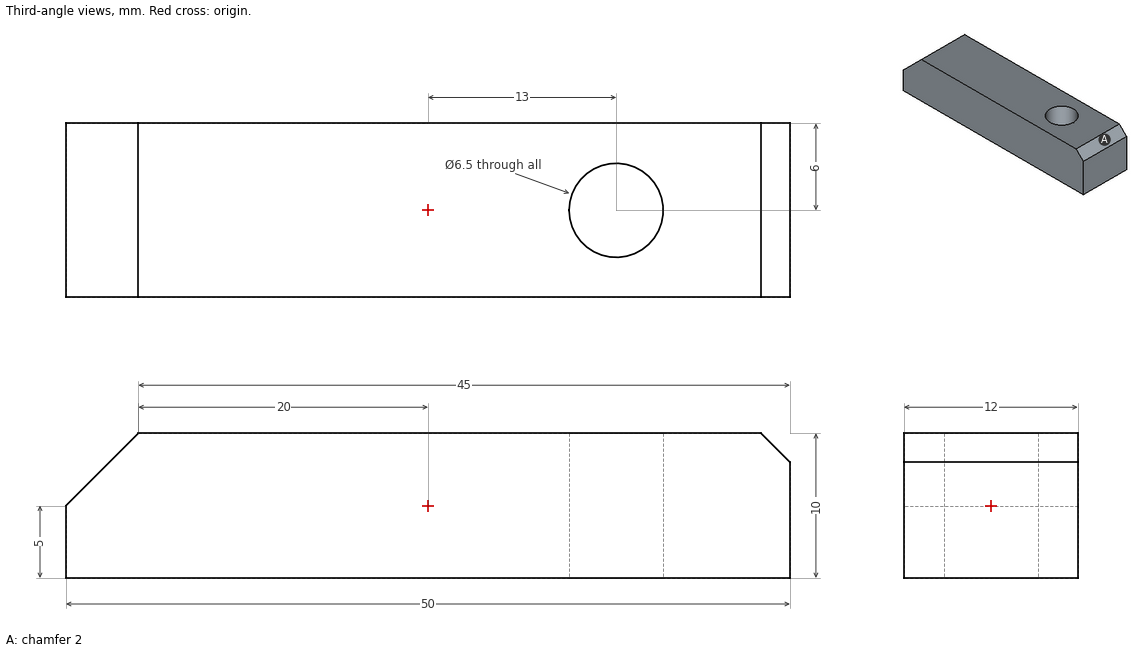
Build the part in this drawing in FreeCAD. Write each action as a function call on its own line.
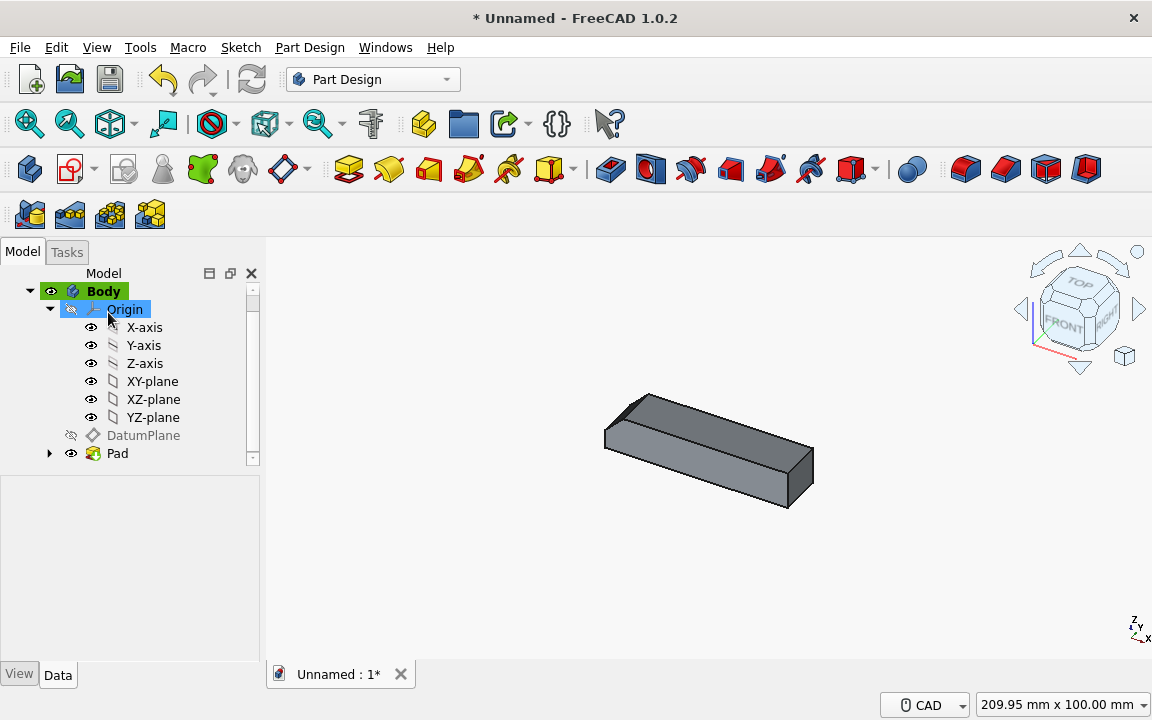
click(30, 124)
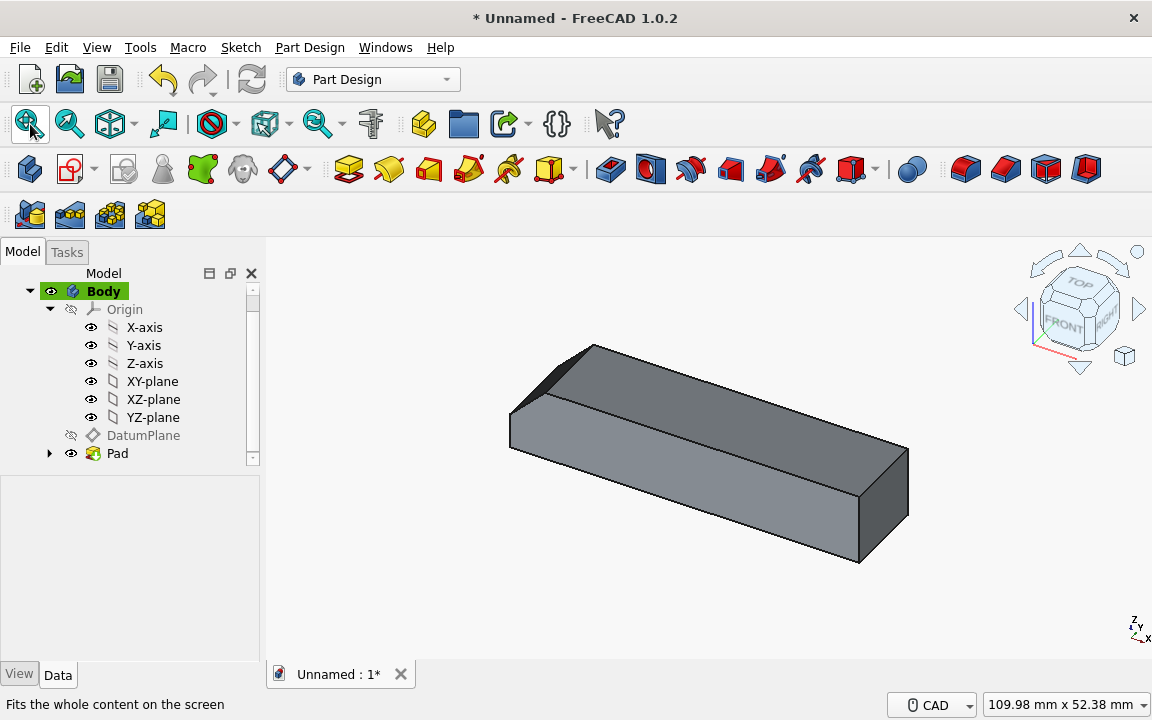
click(816, 449)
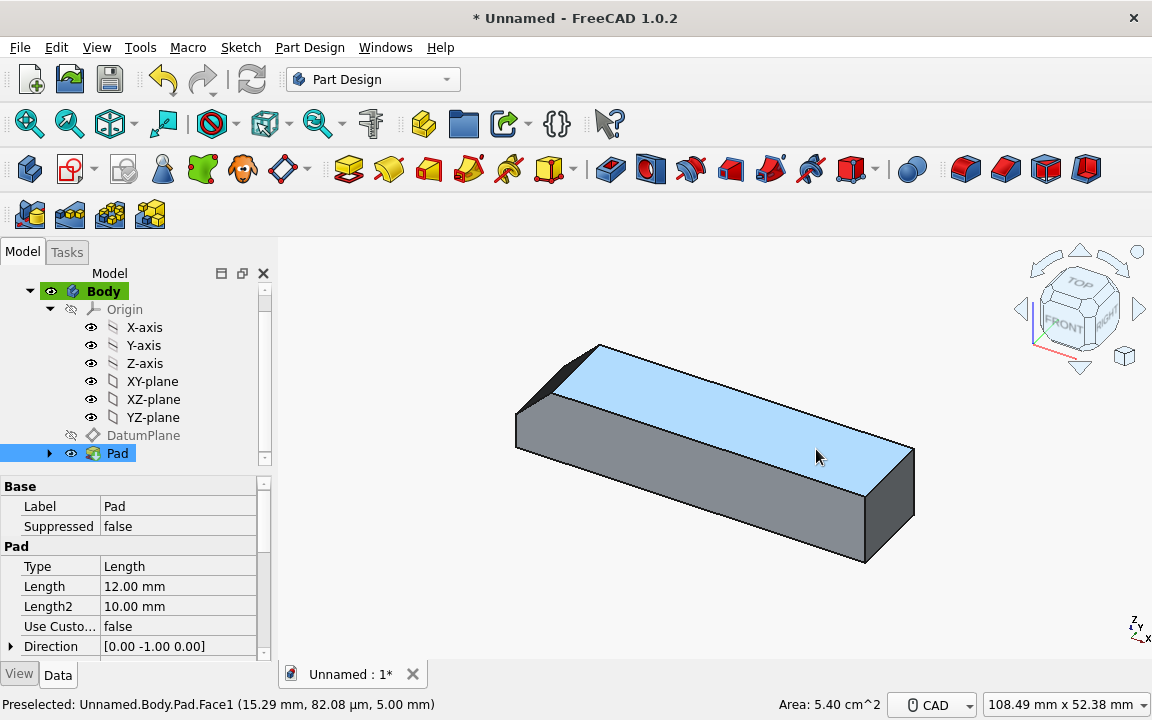
click(70, 170)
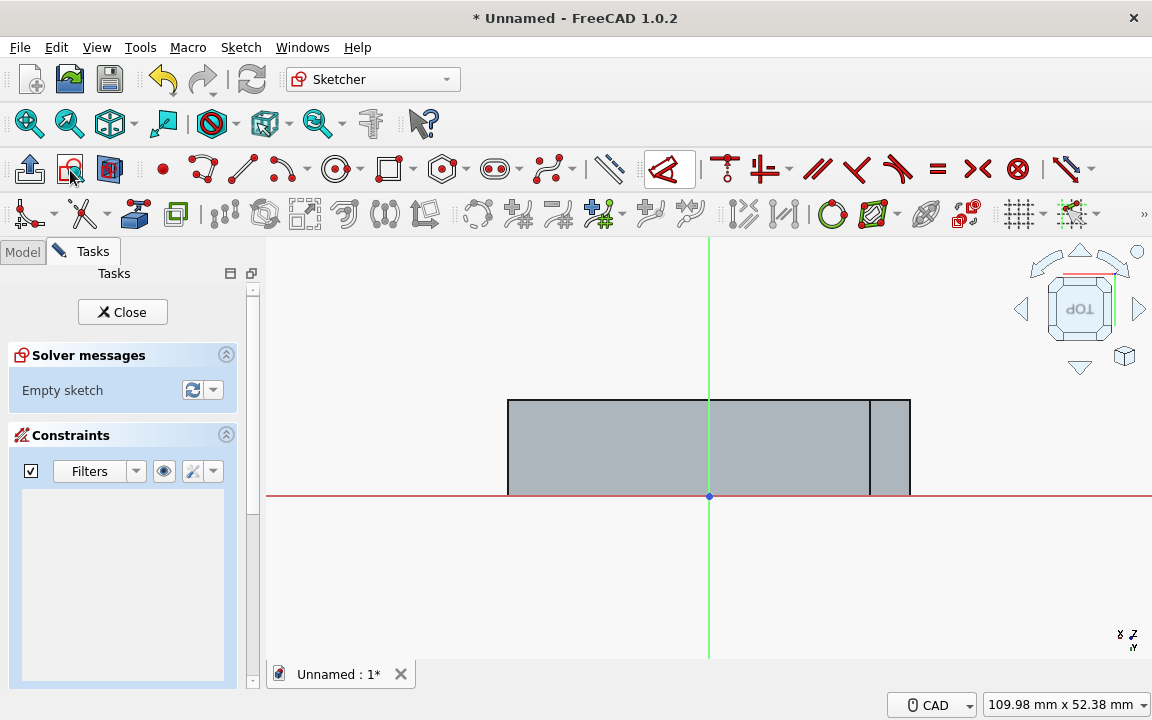
scroll(595, 448, up, 8)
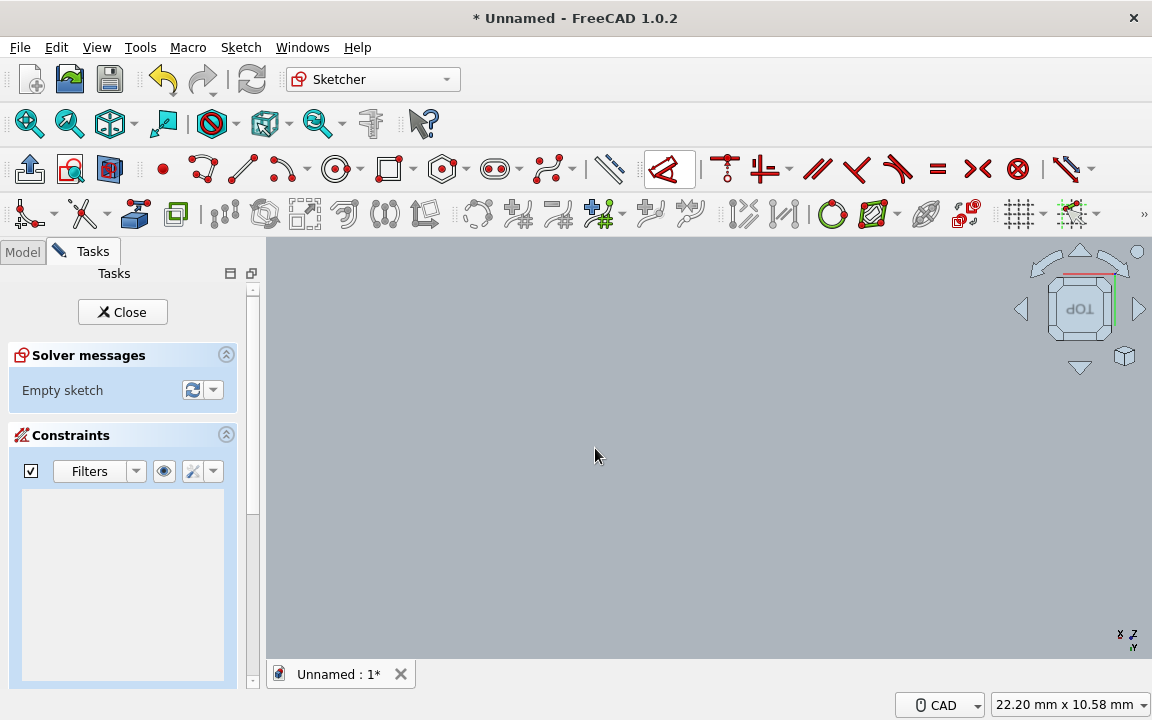
click(336, 170)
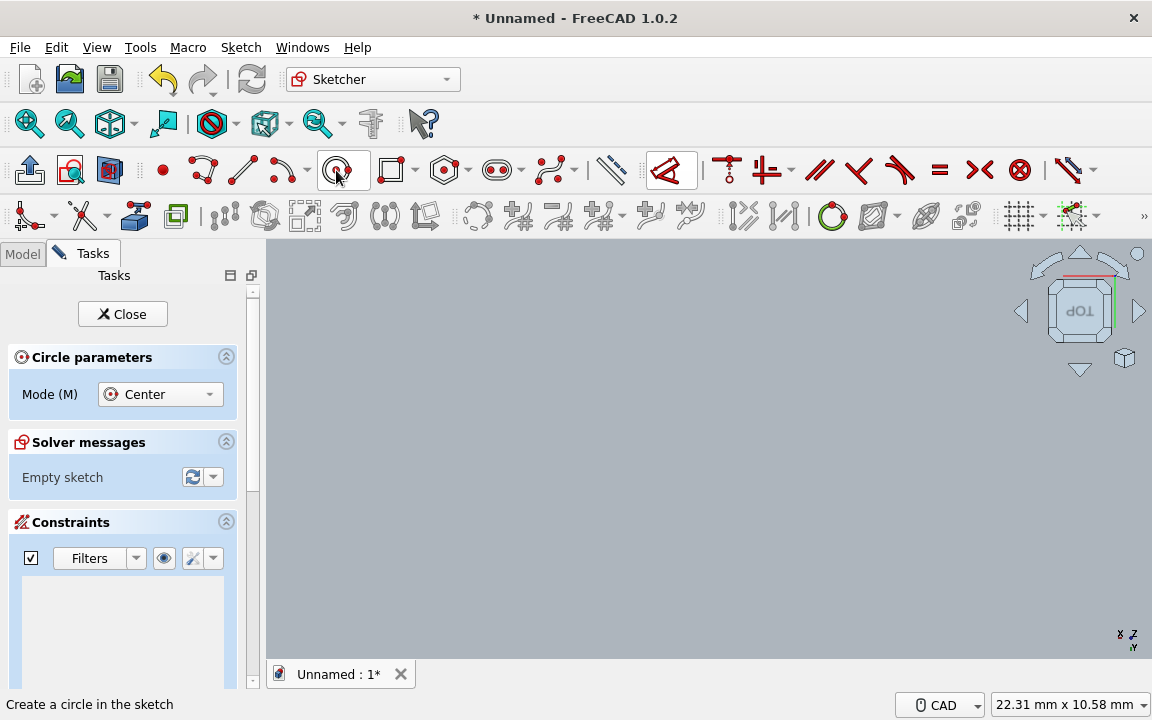
click(640, 447)
click(731, 356)
key(Escape)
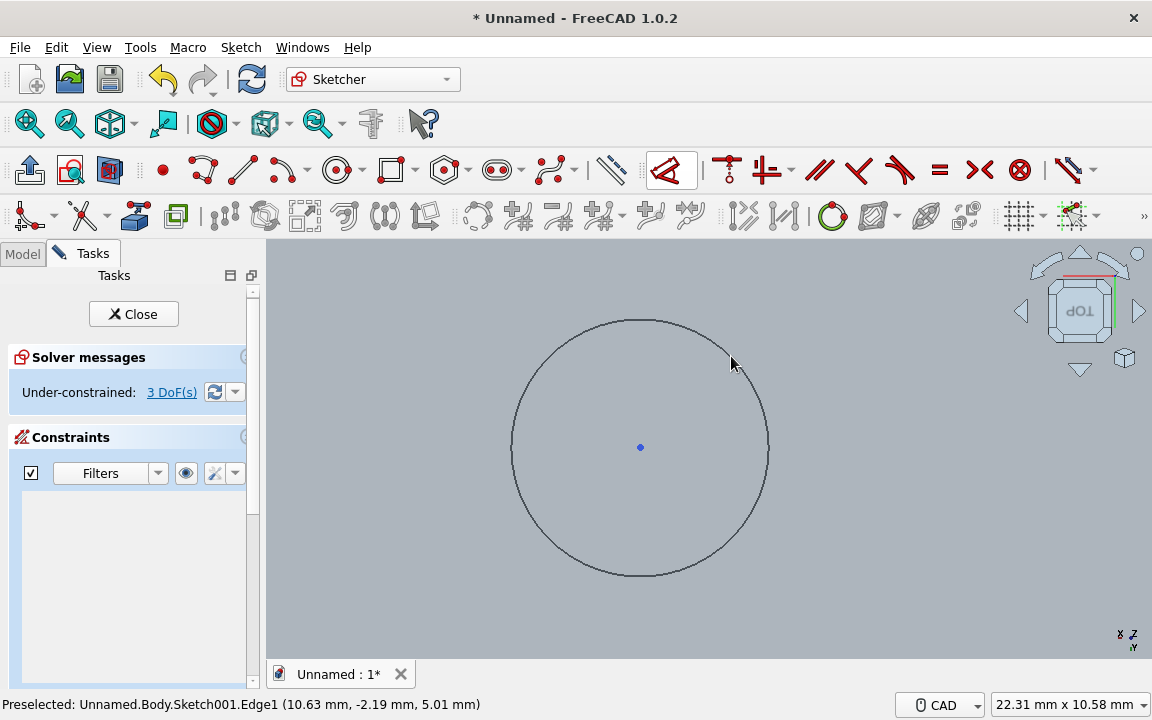
click(731, 357)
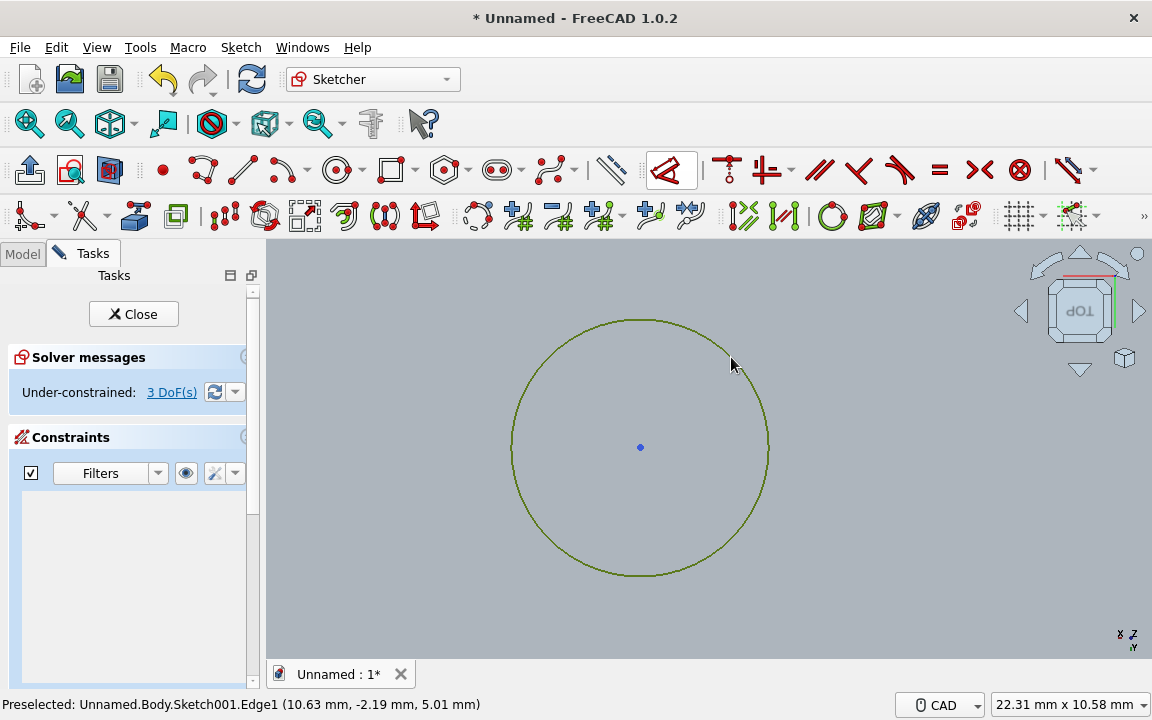
click(692, 170)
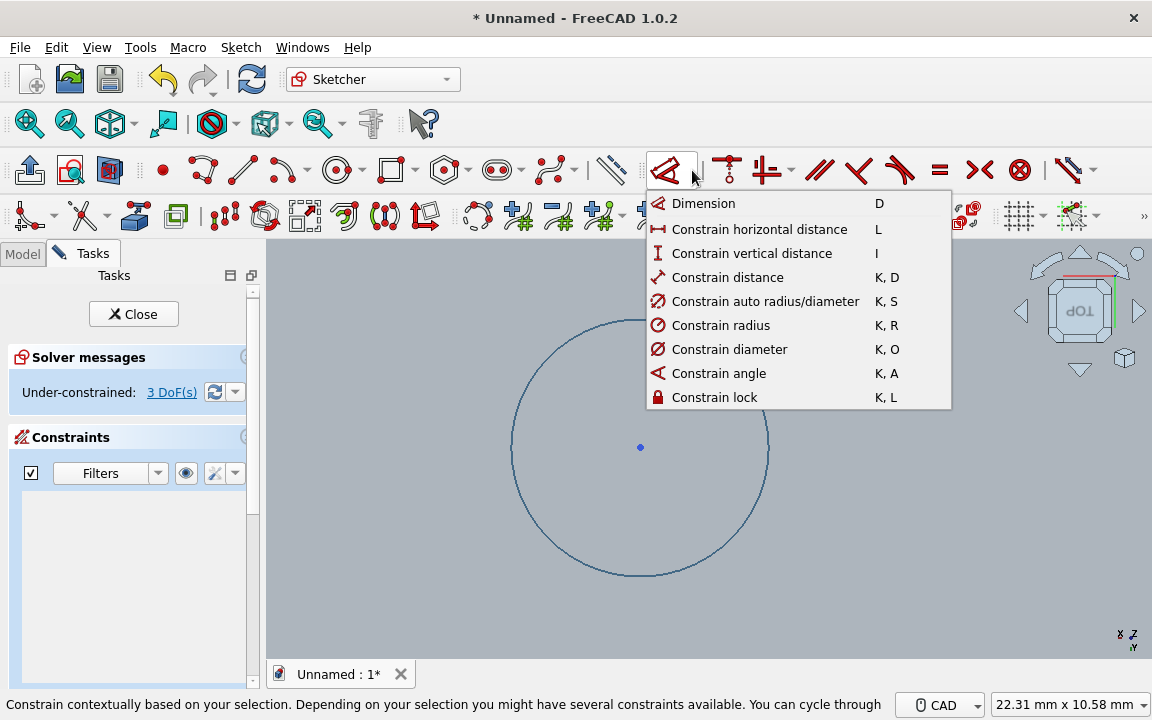
click(799, 349)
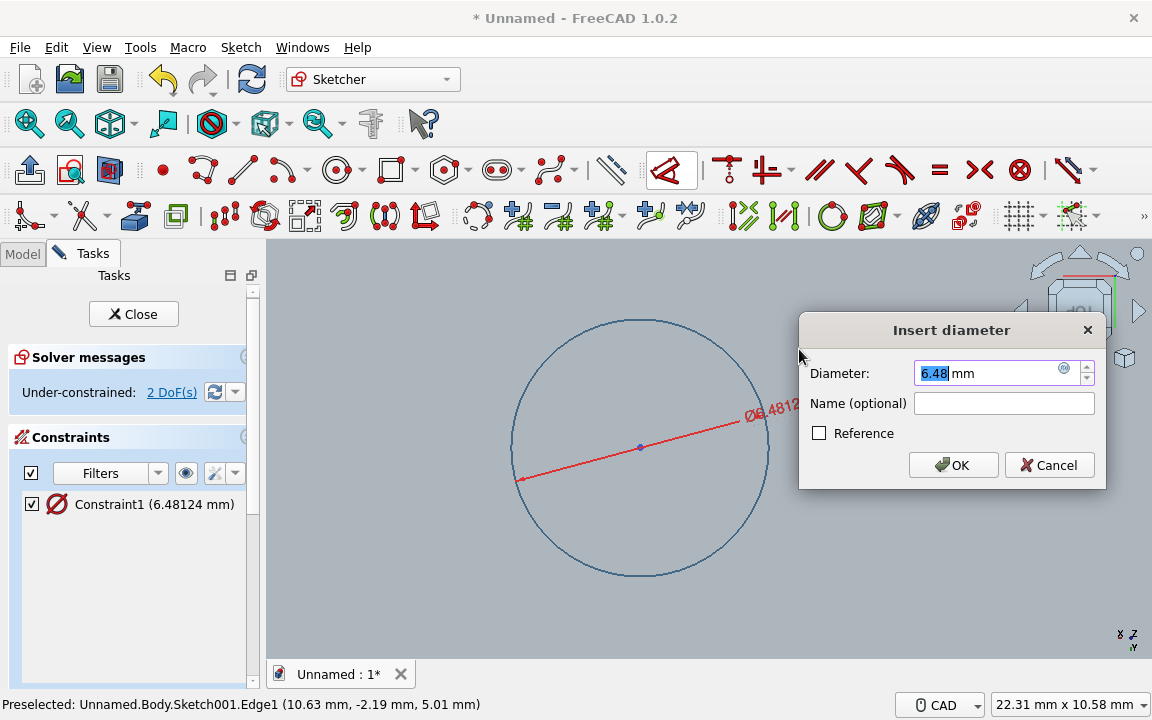
text(6.5)
key(Return)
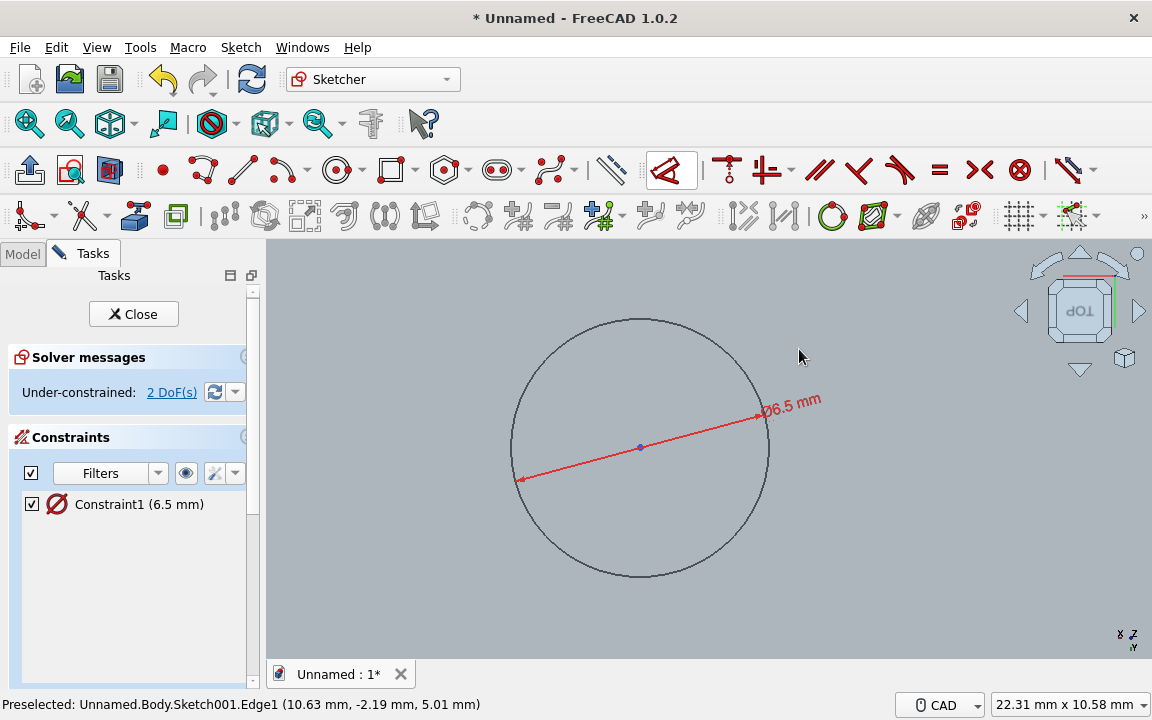
click(640, 448)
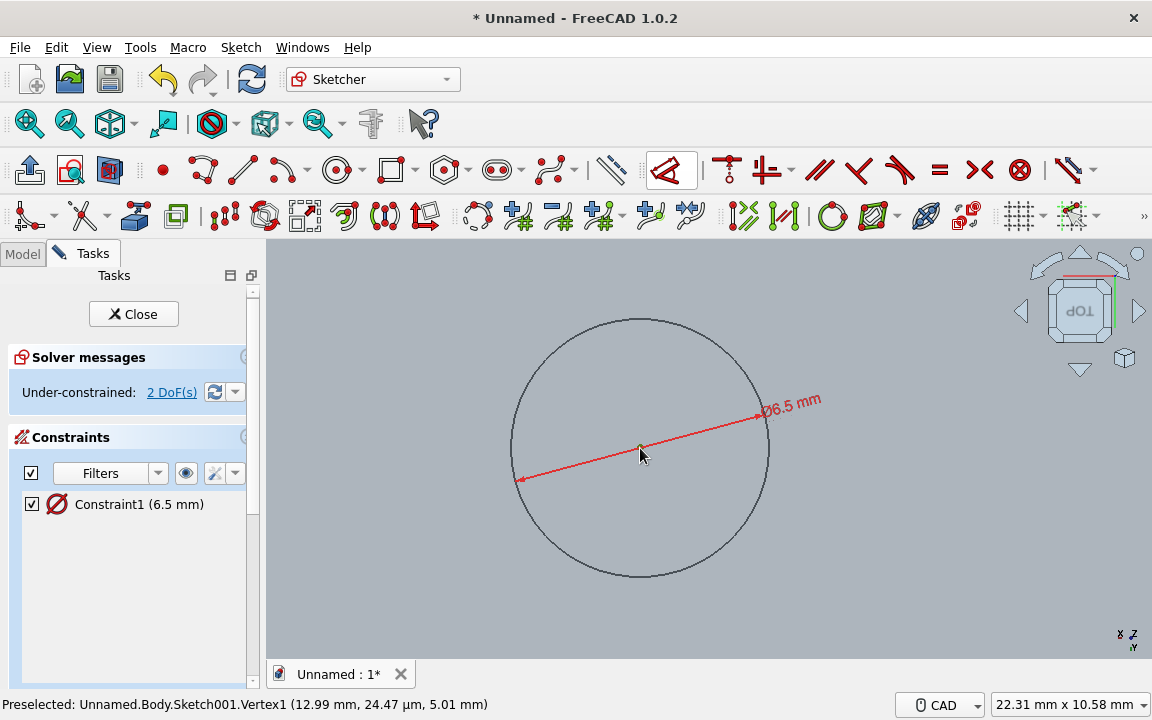
click(692, 170)